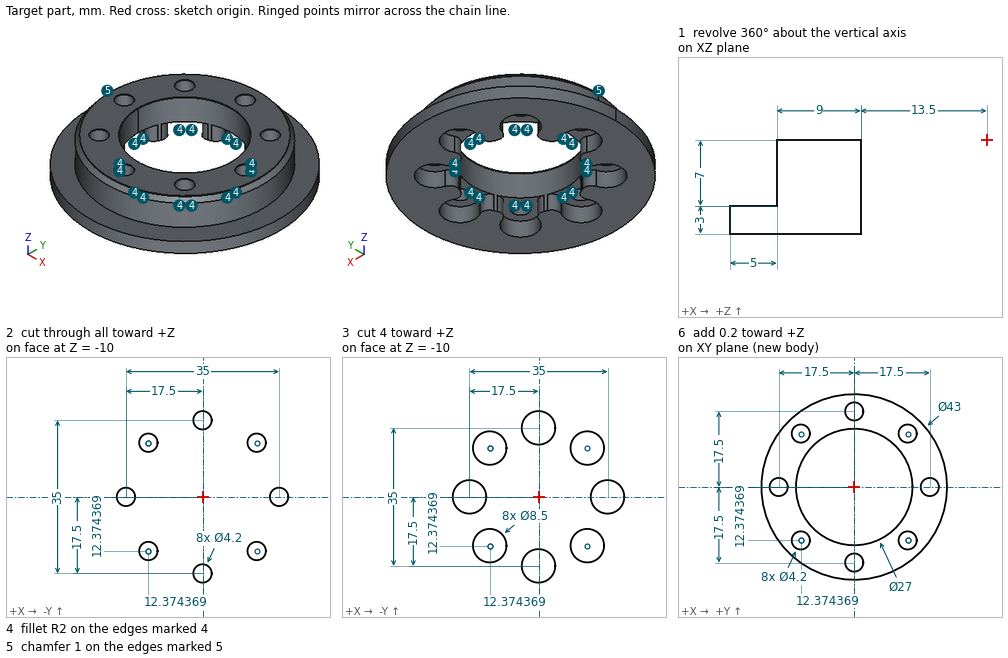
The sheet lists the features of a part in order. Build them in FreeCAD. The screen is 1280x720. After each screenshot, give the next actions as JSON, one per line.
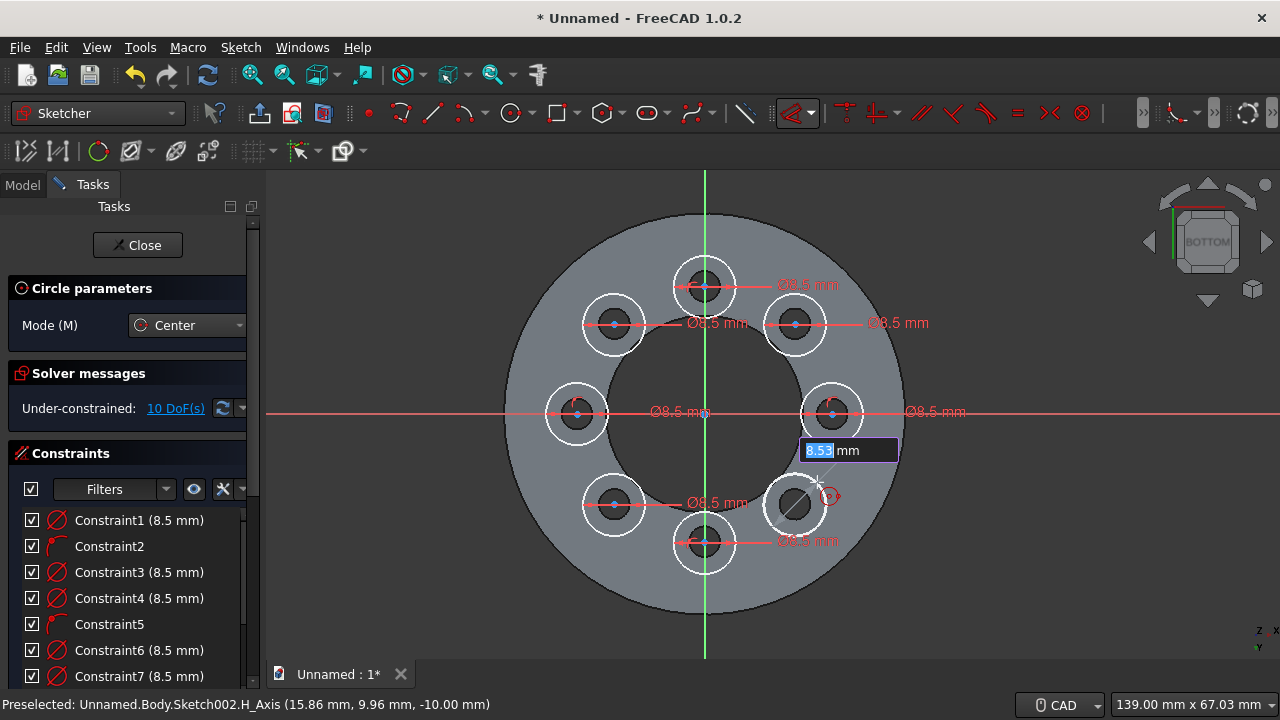
{"action": "type", "text": "8.5"}
{"action": "key", "text": "Return"}
{"action": "key", "text": "Escape"}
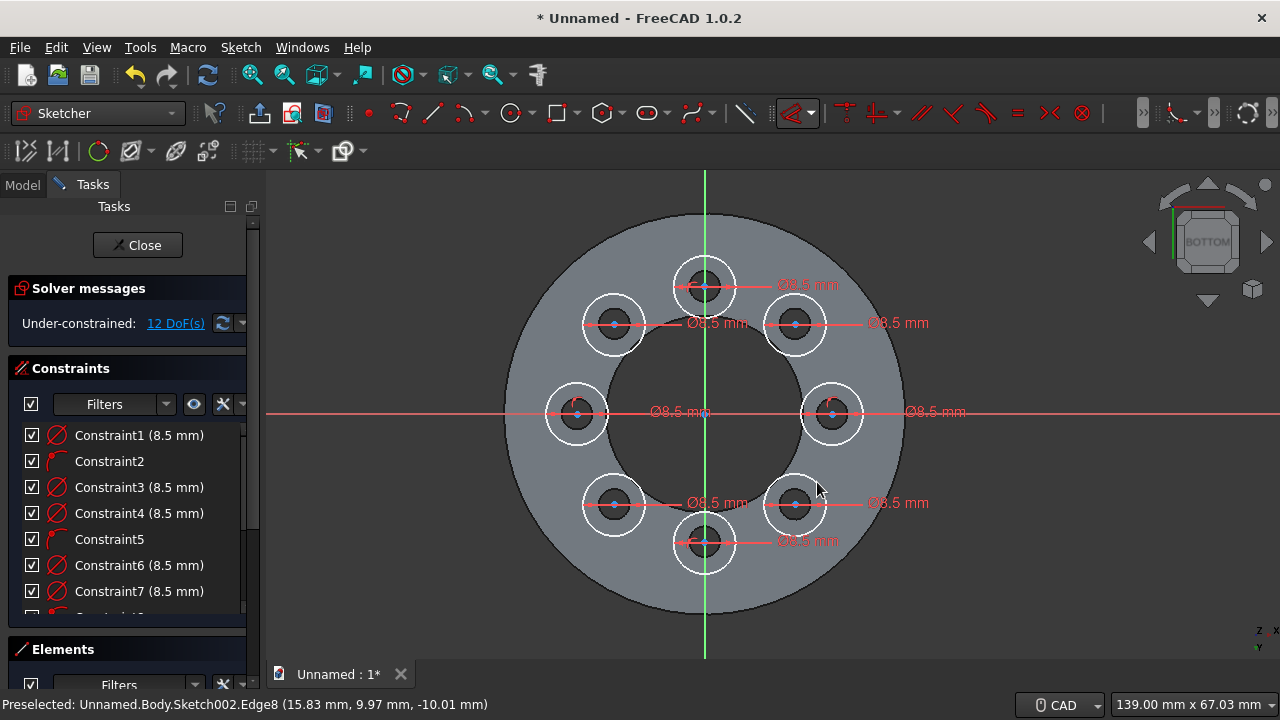
{"action": "left_click", "coordinate": [614, 505]}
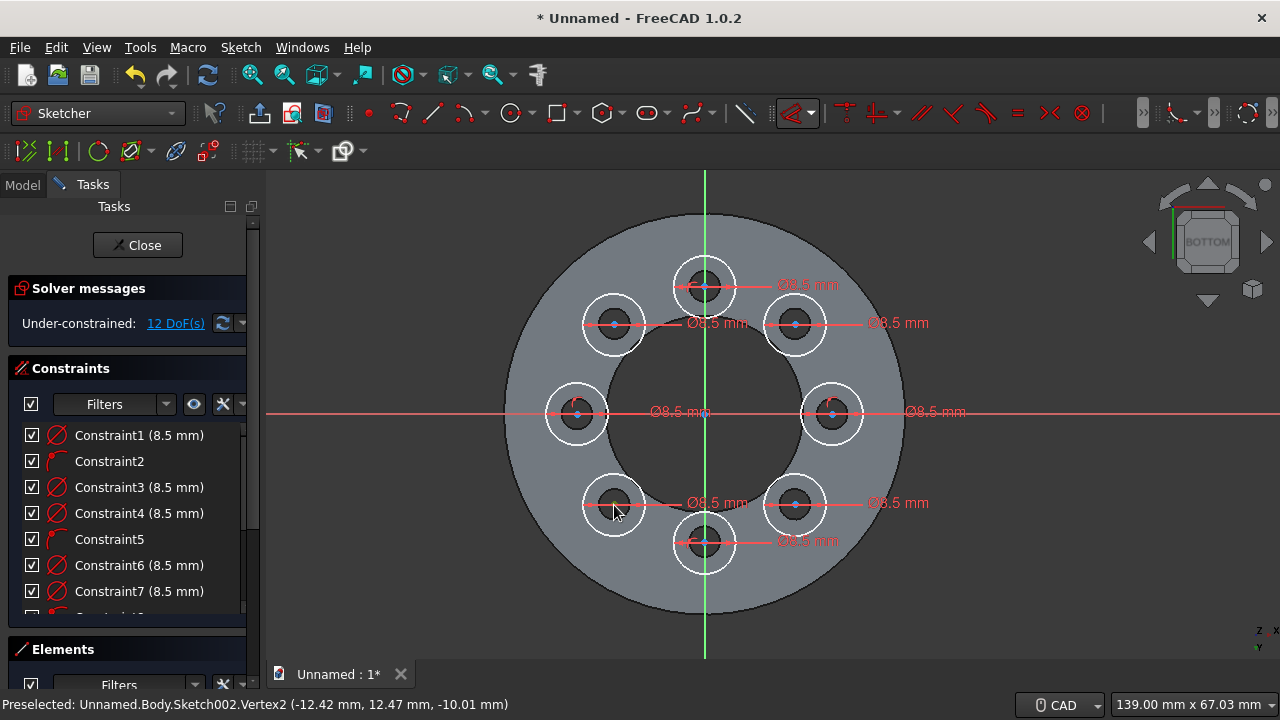
{"action": "left_click", "coordinate": [614, 325]}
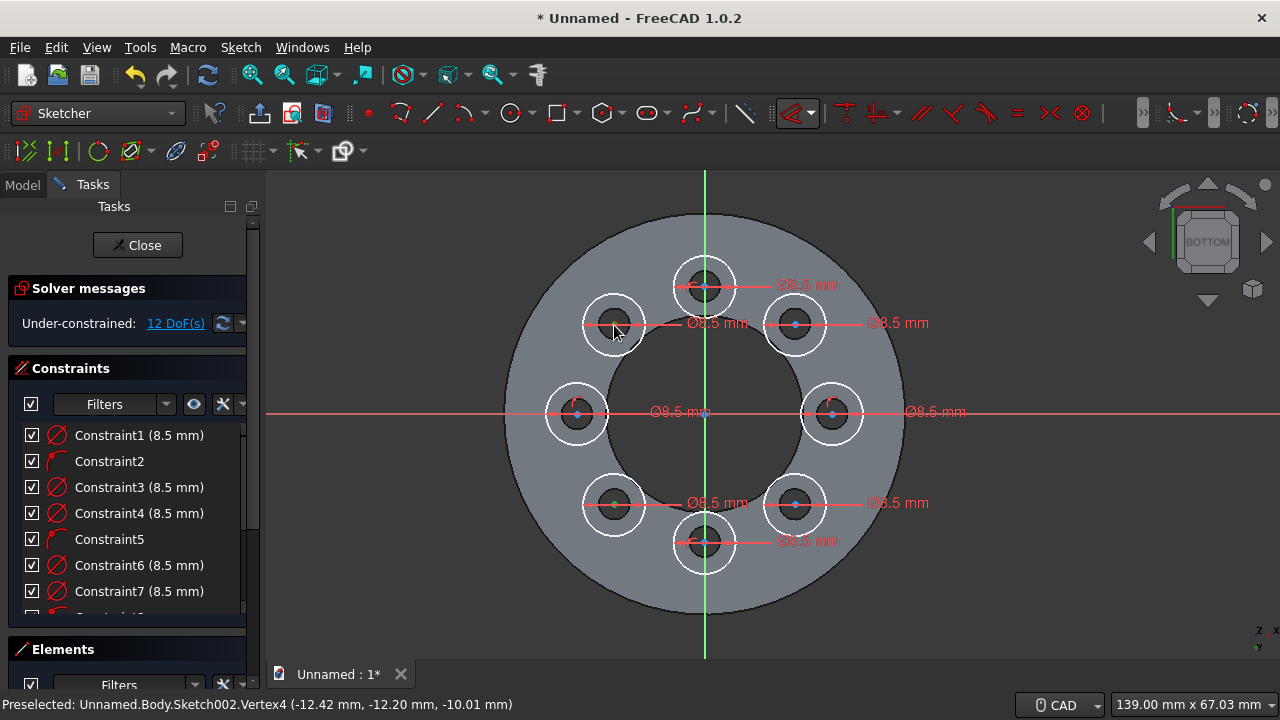
{"action": "left_click", "coordinate": [353, 414]}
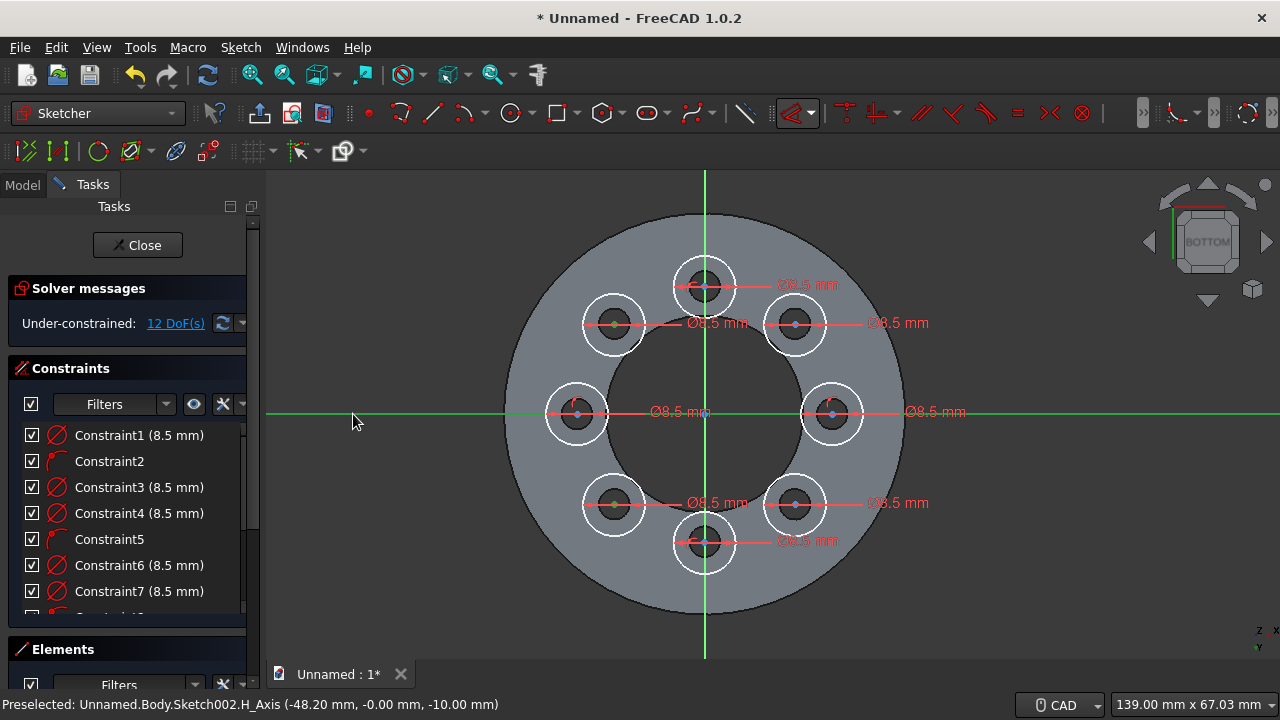
{"action": "key", "text": "s"}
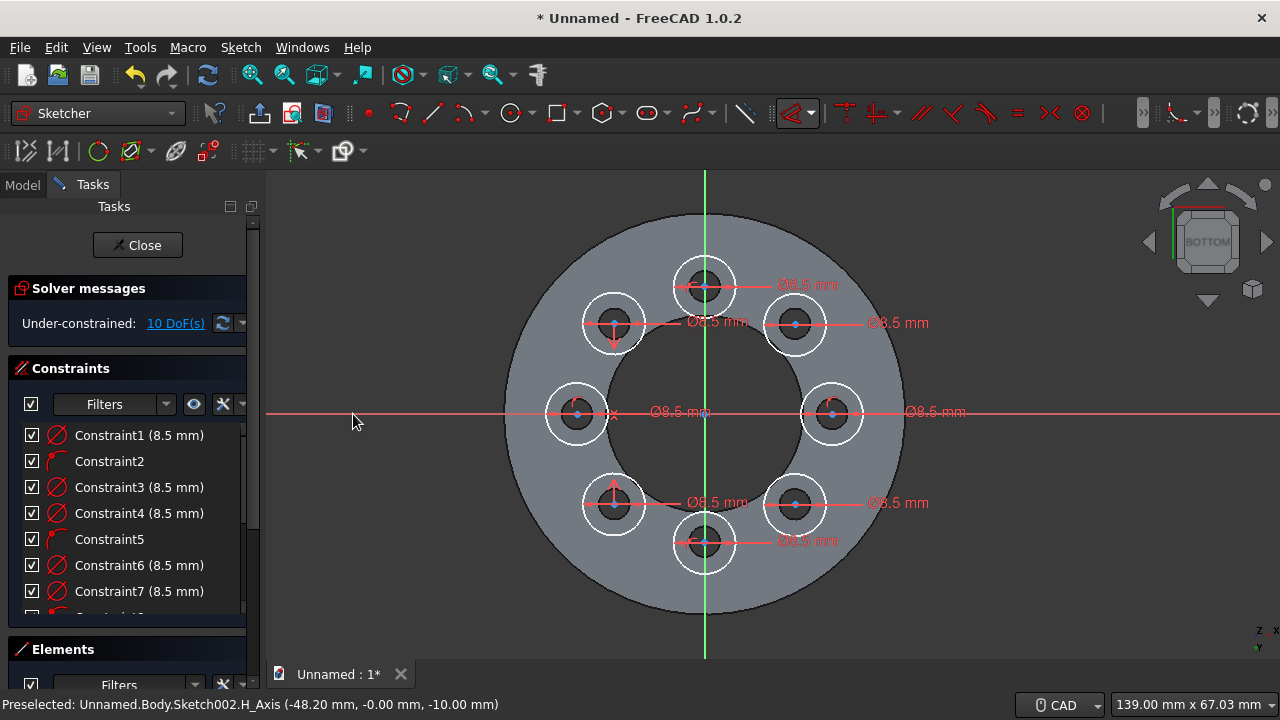
{"action": "left_click", "coordinate": [614, 324]}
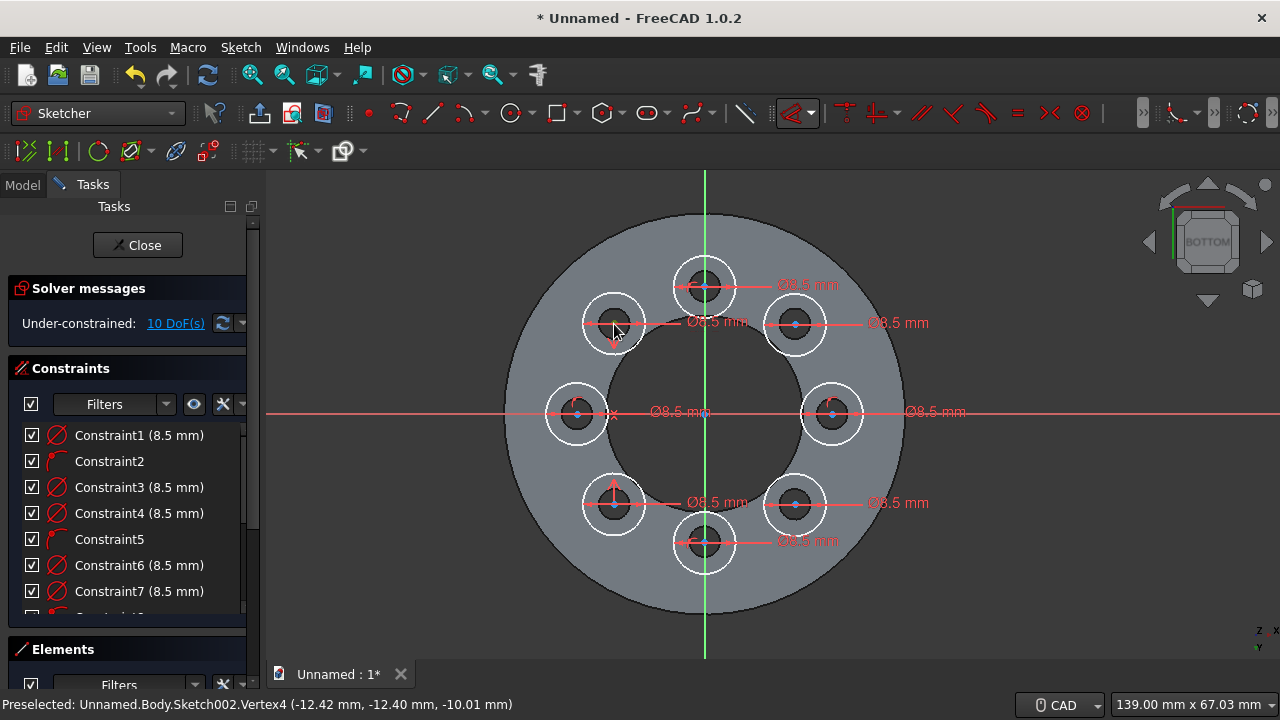
{"action": "left_click", "coordinate": [795, 325]}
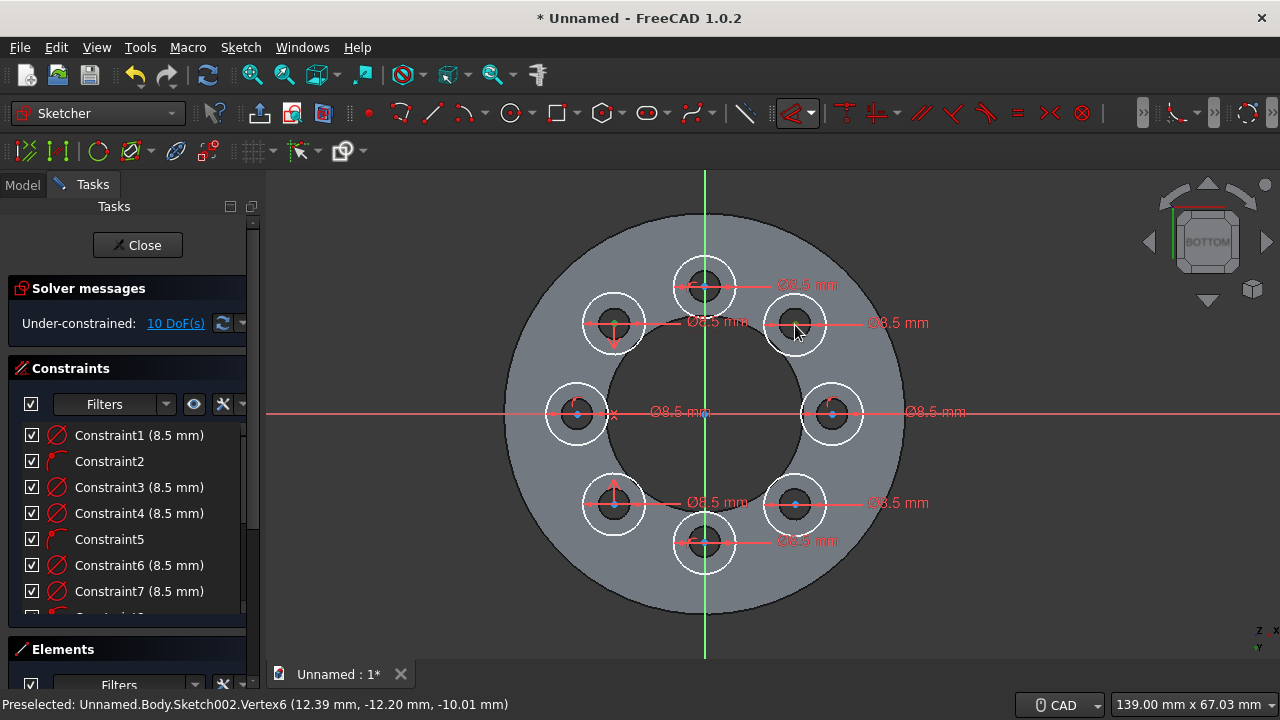
{"action": "left_click", "coordinate": [705, 476]}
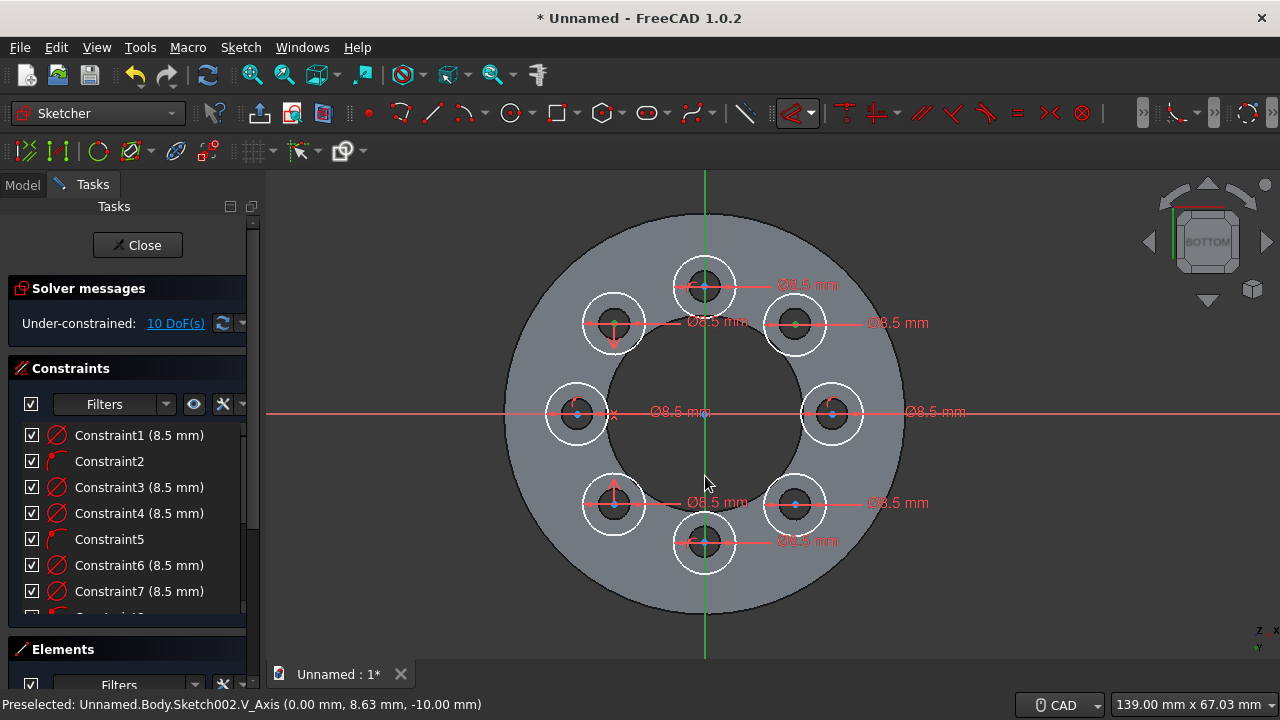
{"action": "key", "text": "s"}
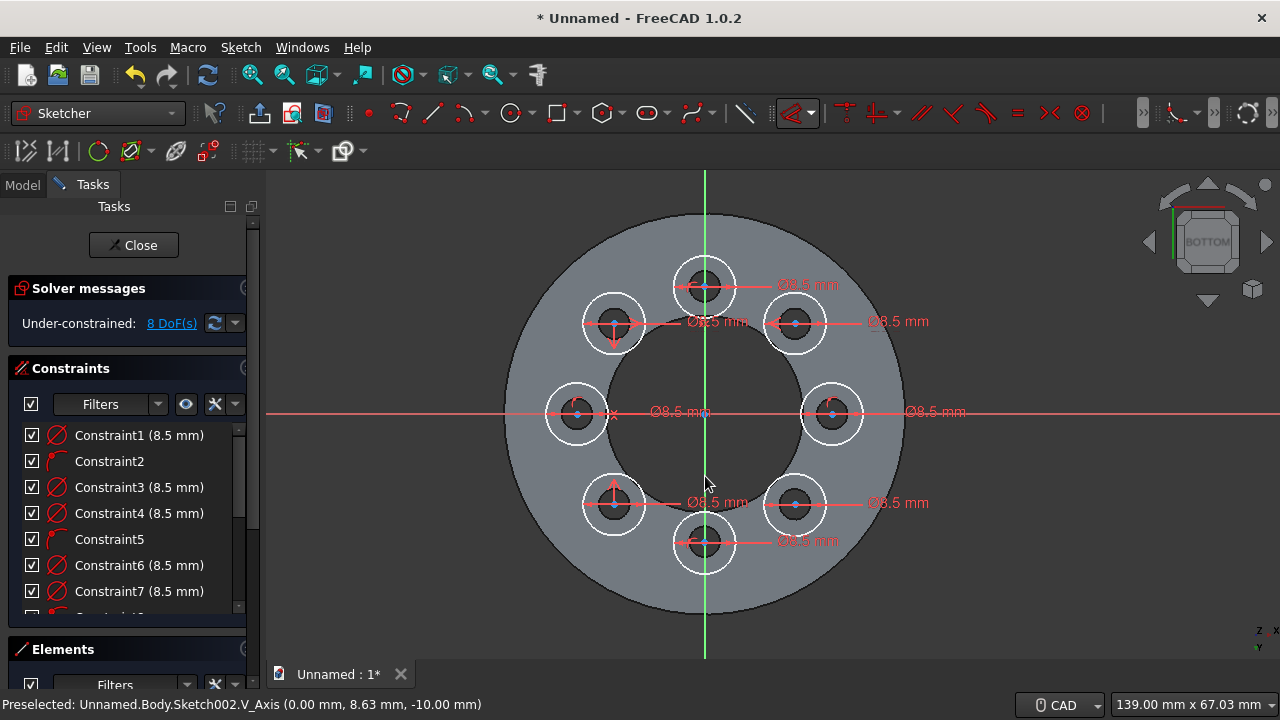
{"action": "left_click", "coordinate": [614, 504]}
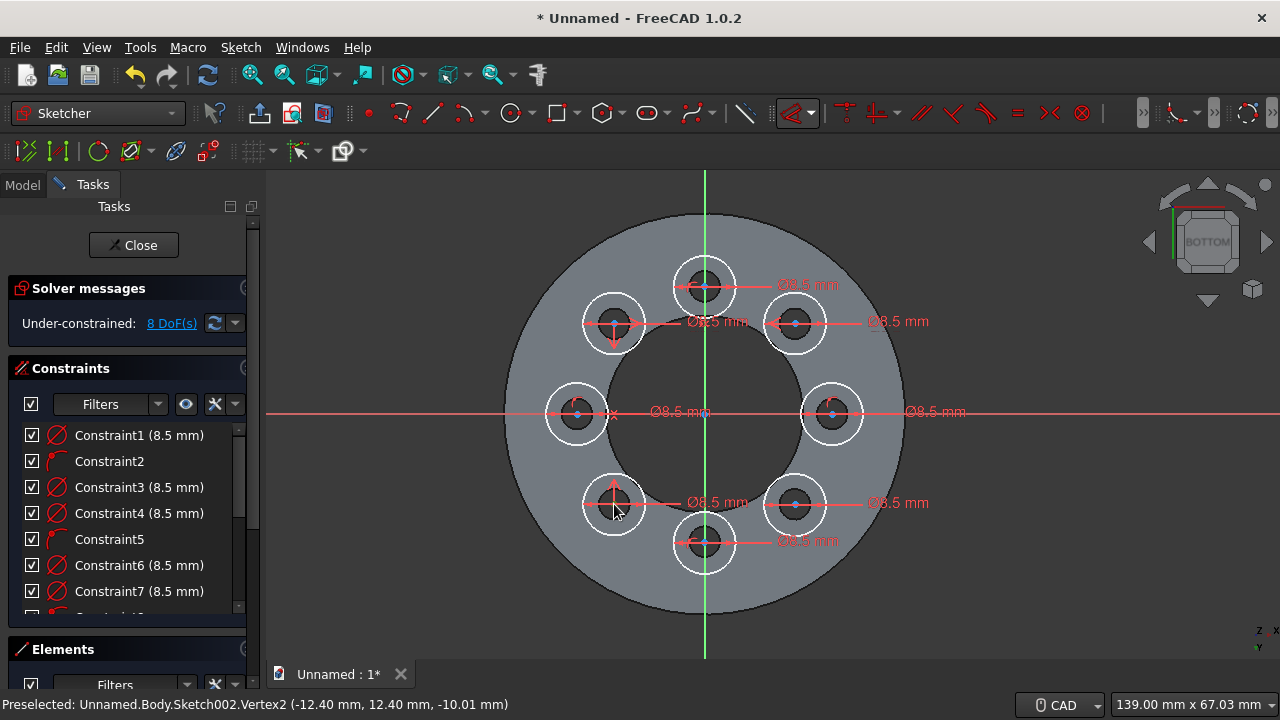
{"action": "left_click", "coordinate": [795, 505]}